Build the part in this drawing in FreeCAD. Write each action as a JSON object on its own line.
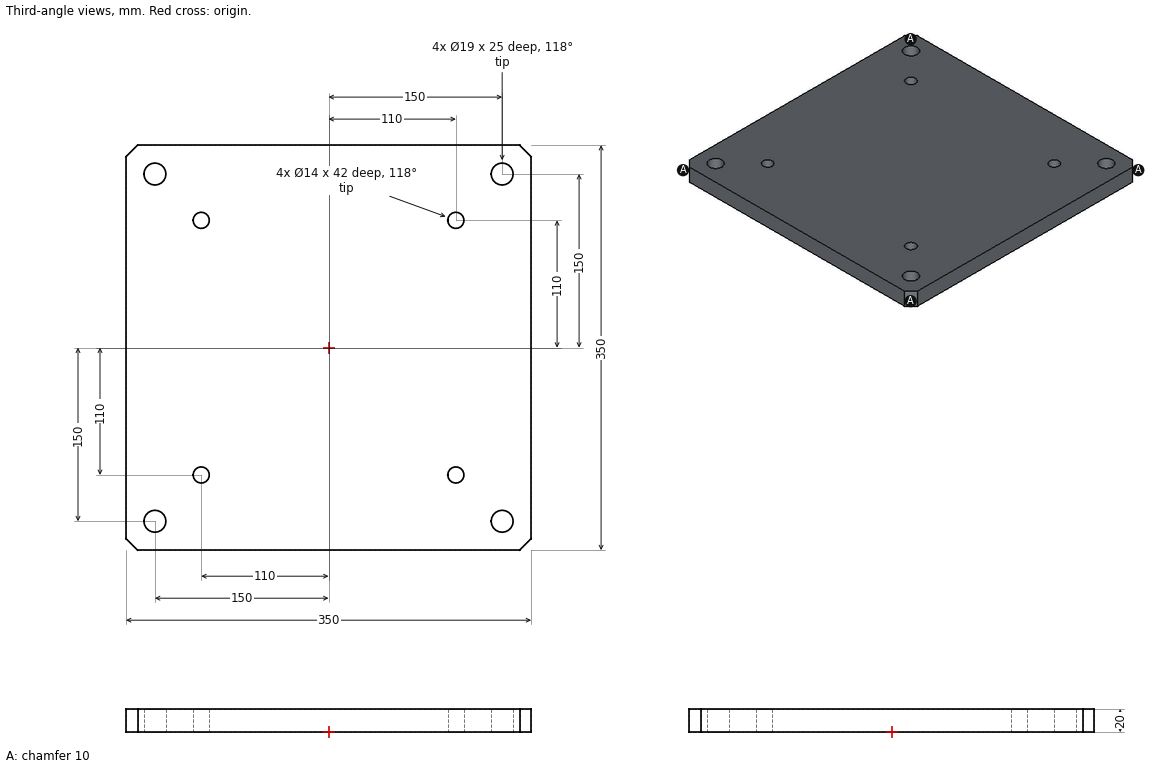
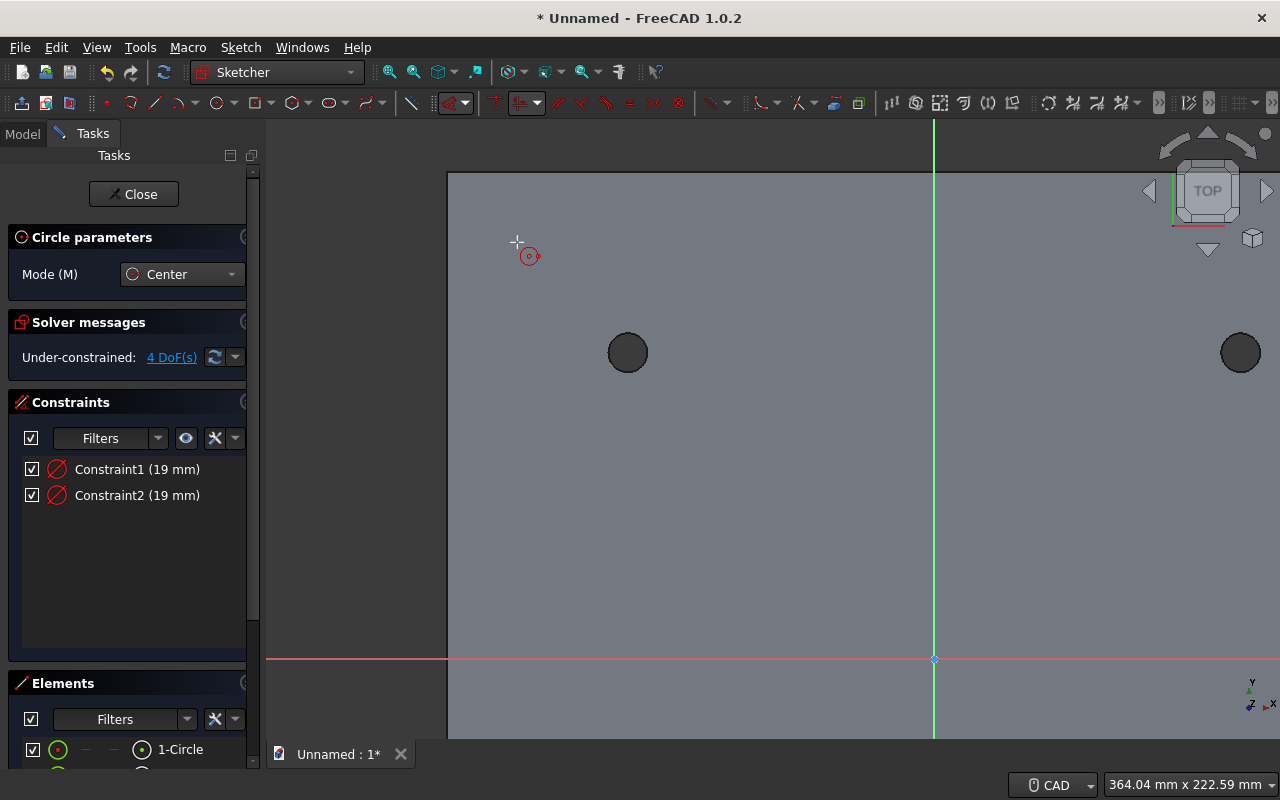
{"action": "left_click", "coordinate": [517, 241]}
{"action": "mouse_move", "coordinate": [535, 223]}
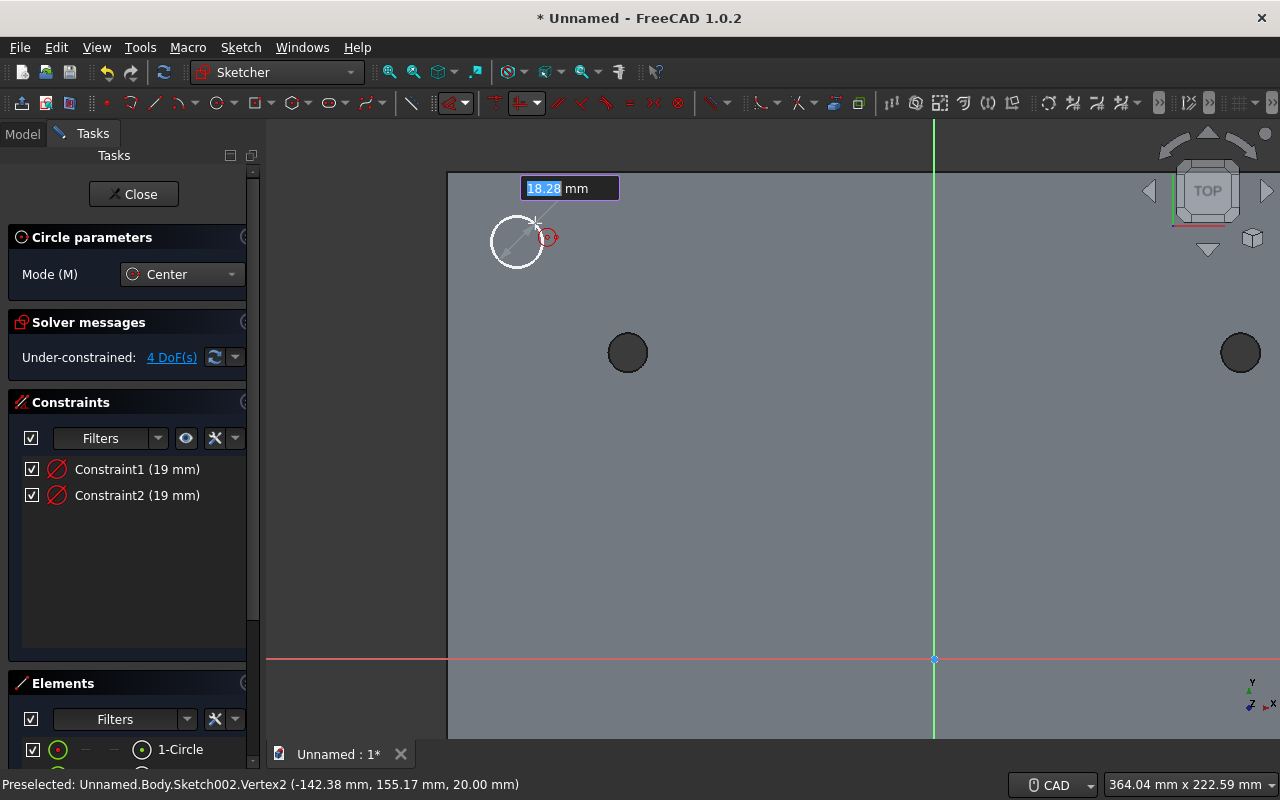
{"action": "type", "text": "19"}
{"action": "key", "text": "Return"}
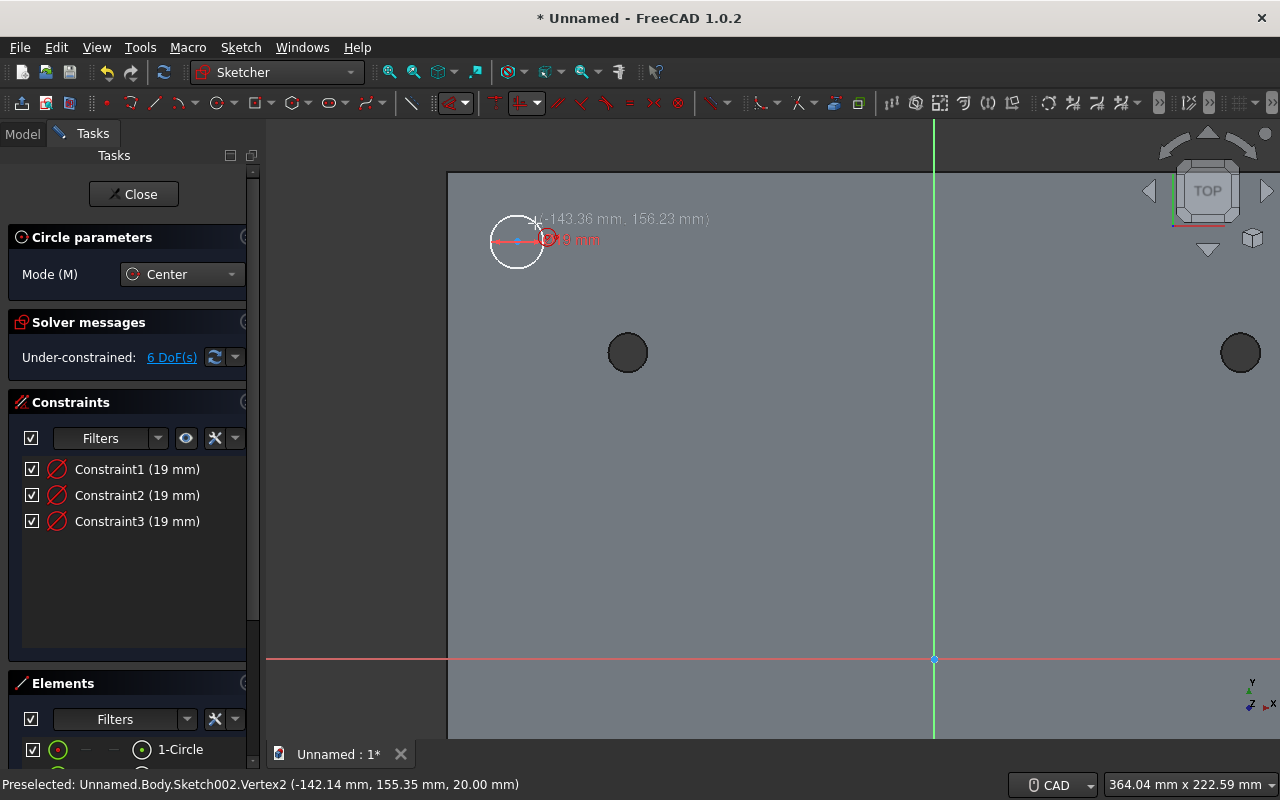
{"action": "scroll", "coordinate": [517, 241], "scroll_direction": "down", "scroll_amount": 4}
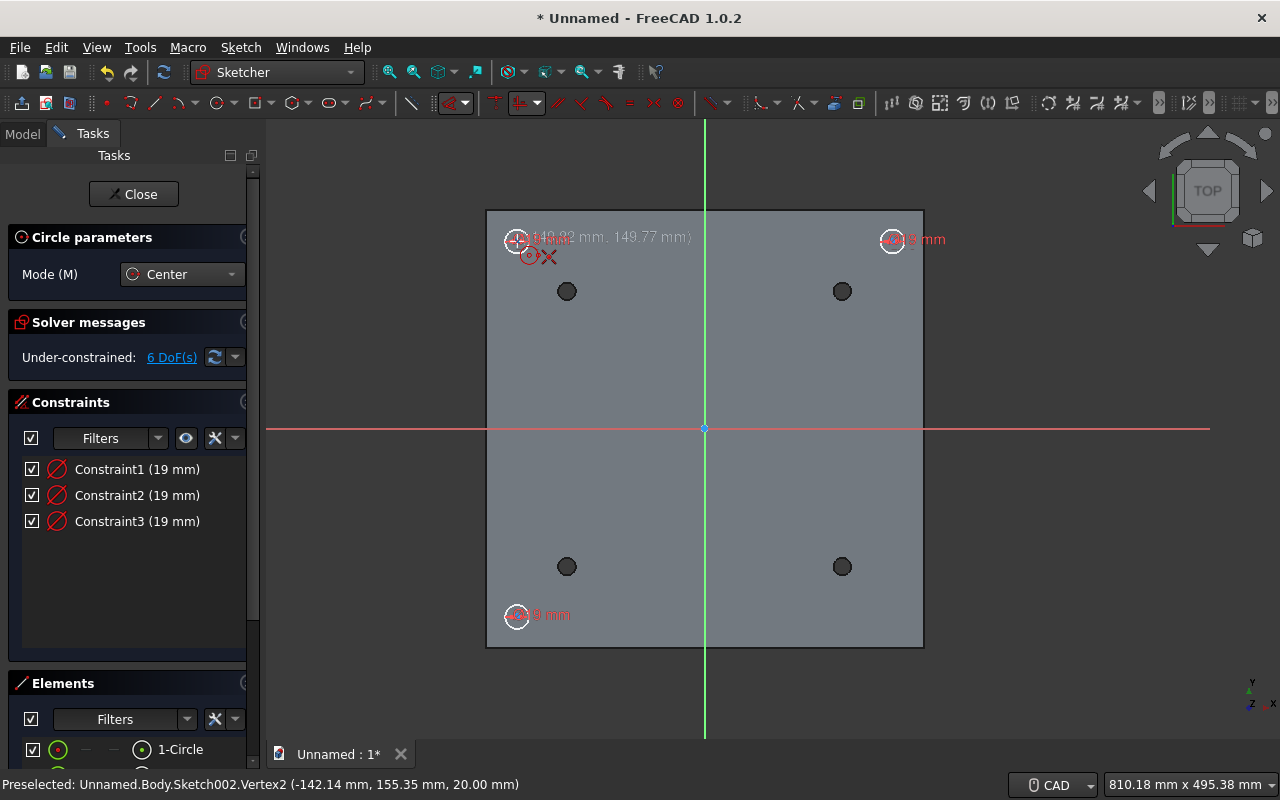
{"action": "scroll", "coordinate": [892, 617], "scroll_direction": "up", "scroll_amount": 4}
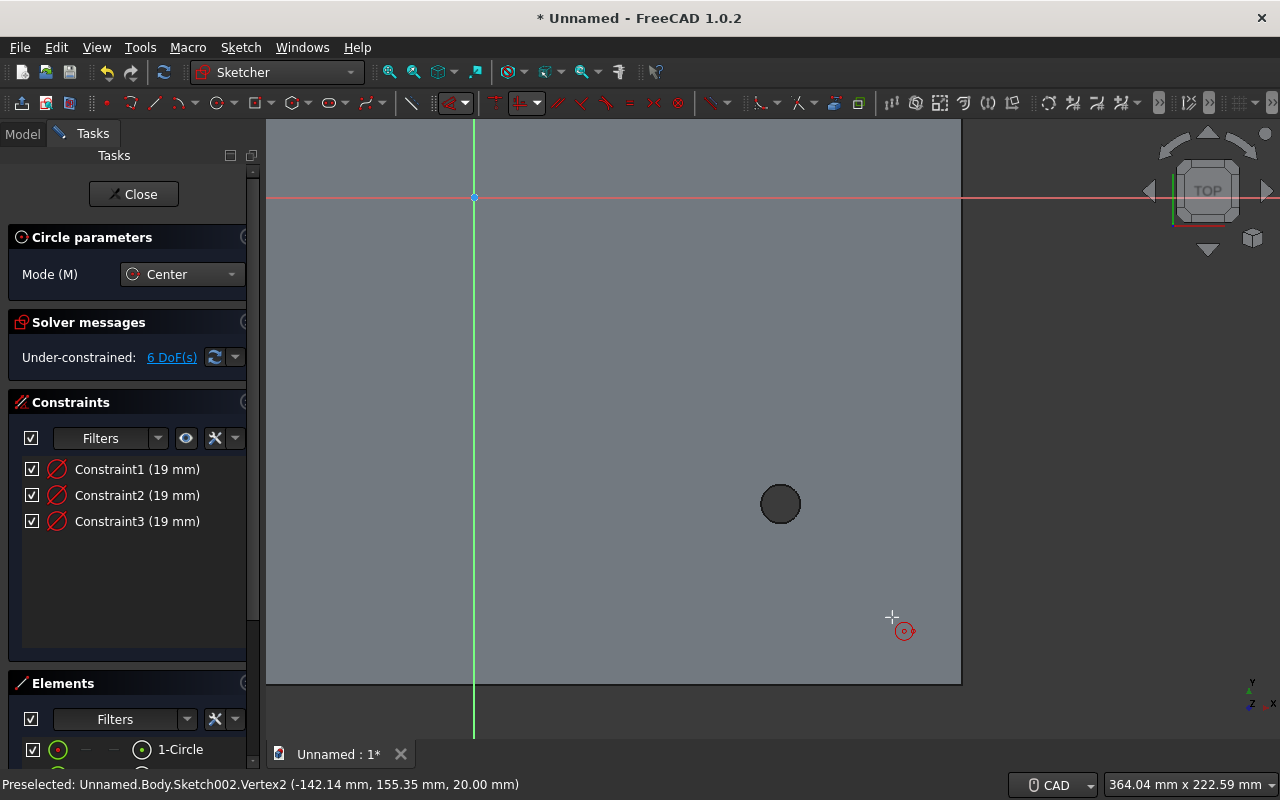
{"action": "left_click", "coordinate": [892, 615]}
{"action": "mouse_move", "coordinate": [911, 597]}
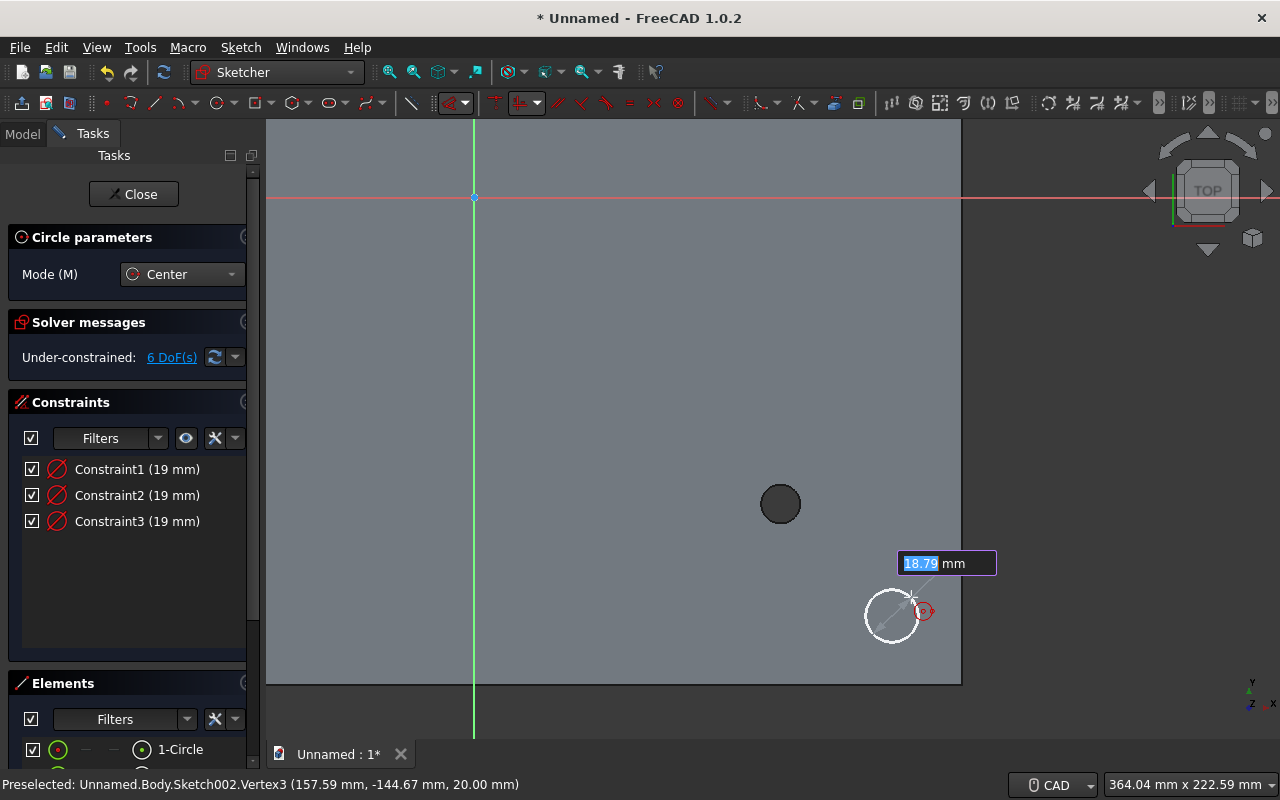
{"action": "type", "text": "19"}
{"action": "key", "text": "Return"}
{"action": "key", "text": "Escape"}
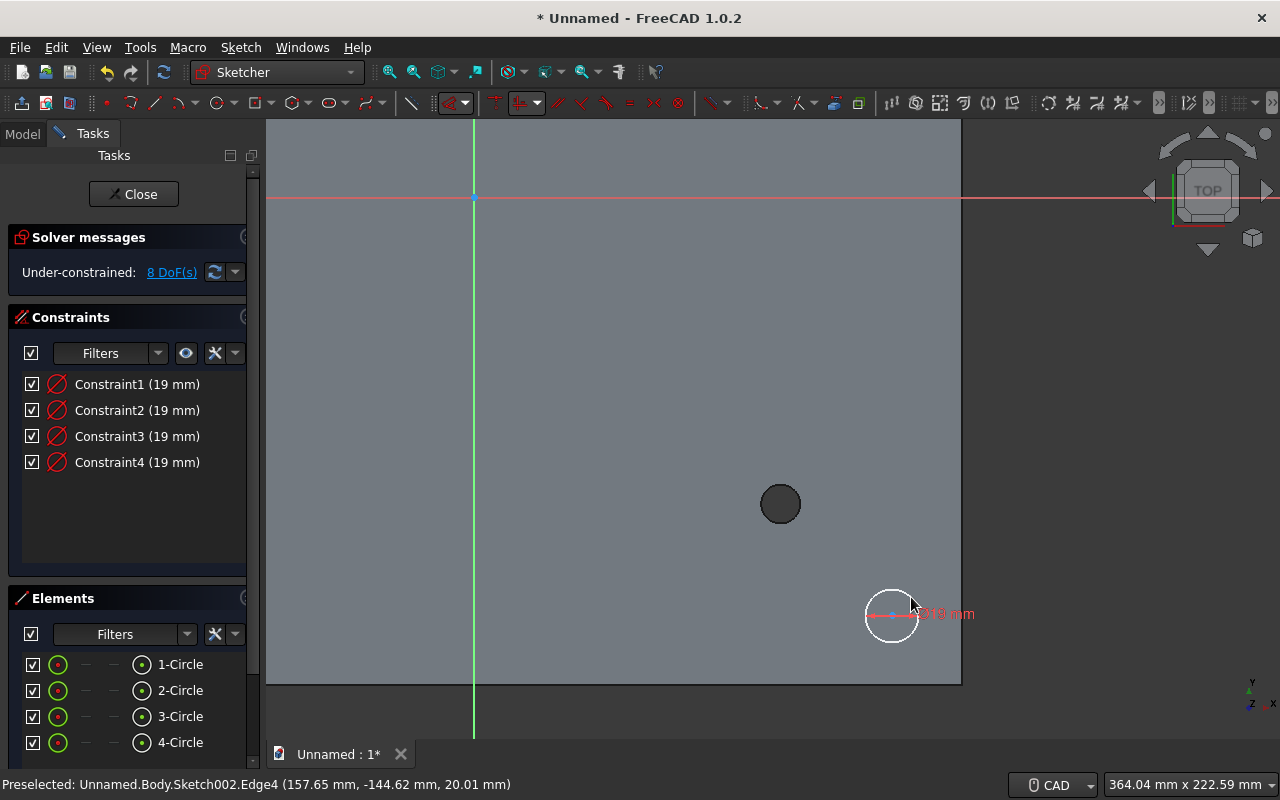
{"action": "scroll", "coordinate": [892, 618], "scroll_direction": "down", "scroll_amount": 4}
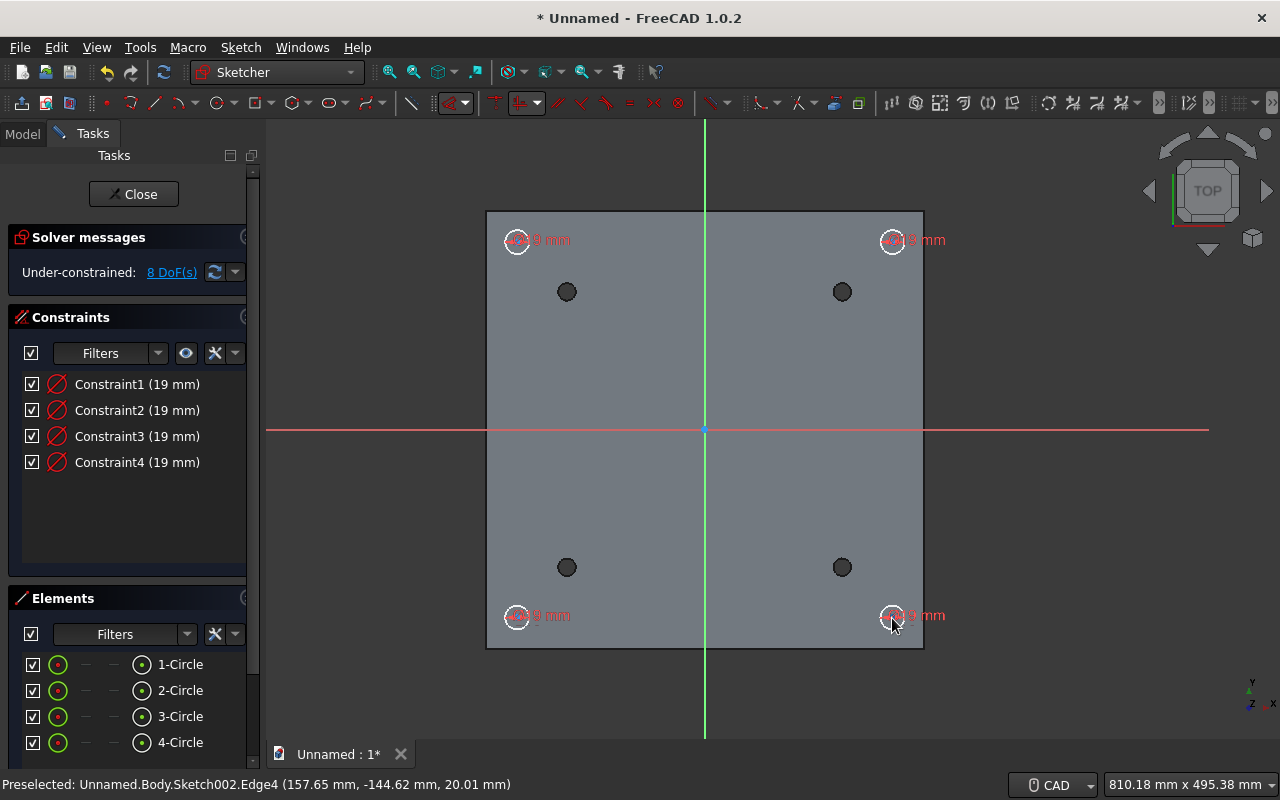
{"action": "left_click", "coordinate": [517, 618]}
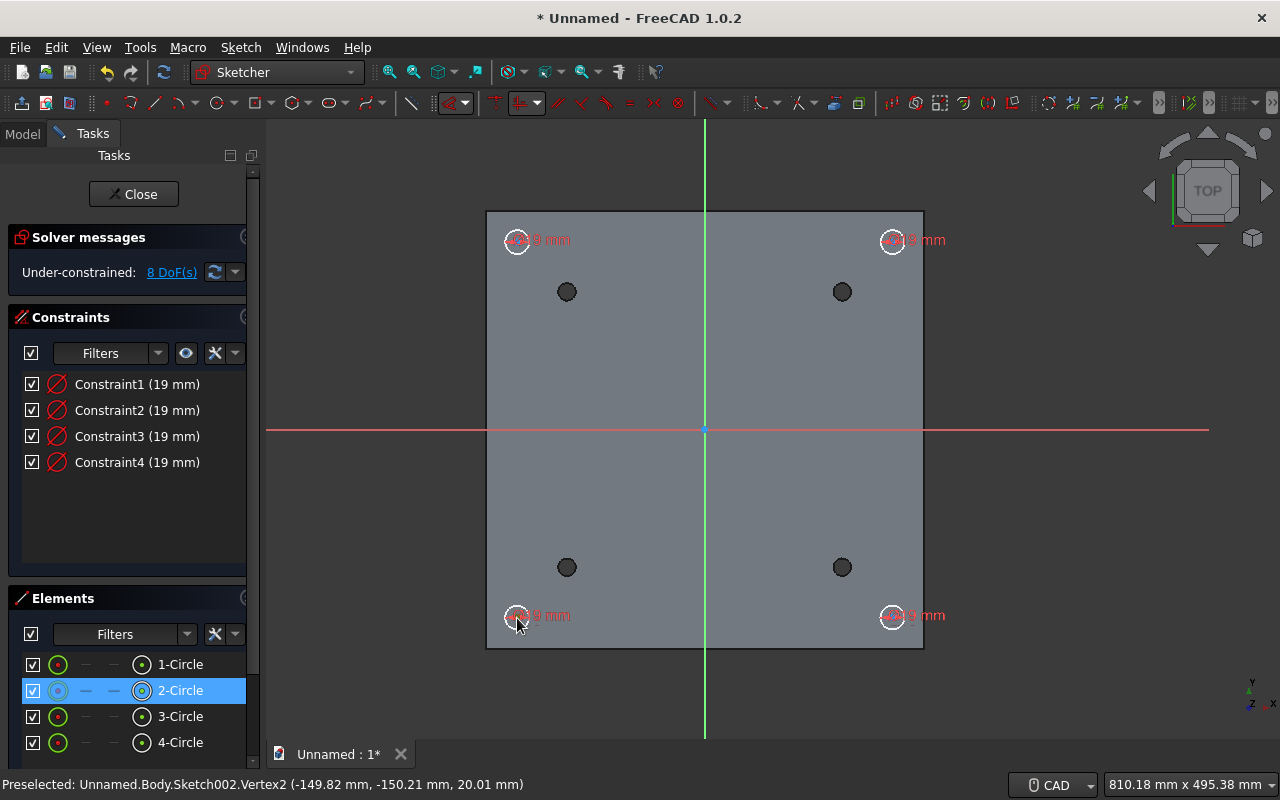
{"action": "left_click", "coordinate": [517, 242]}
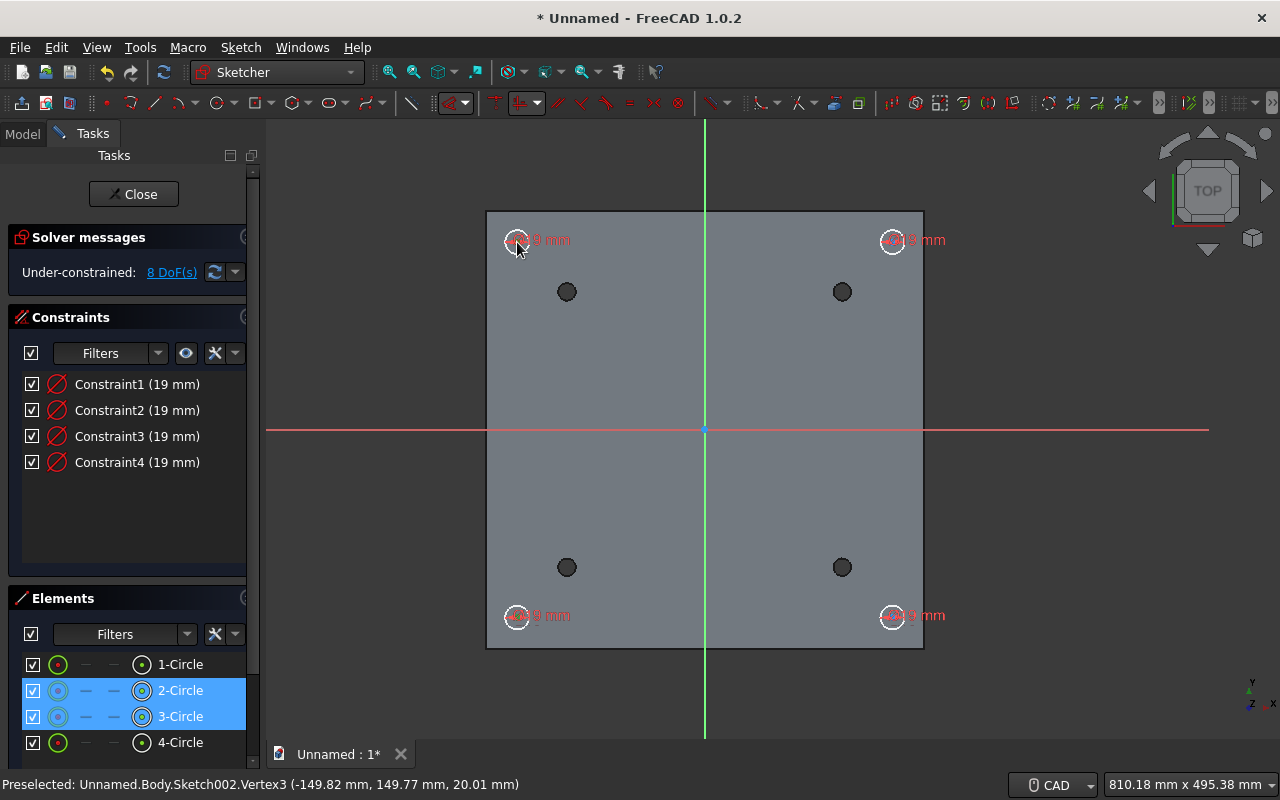
{"action": "key", "text": "v"}